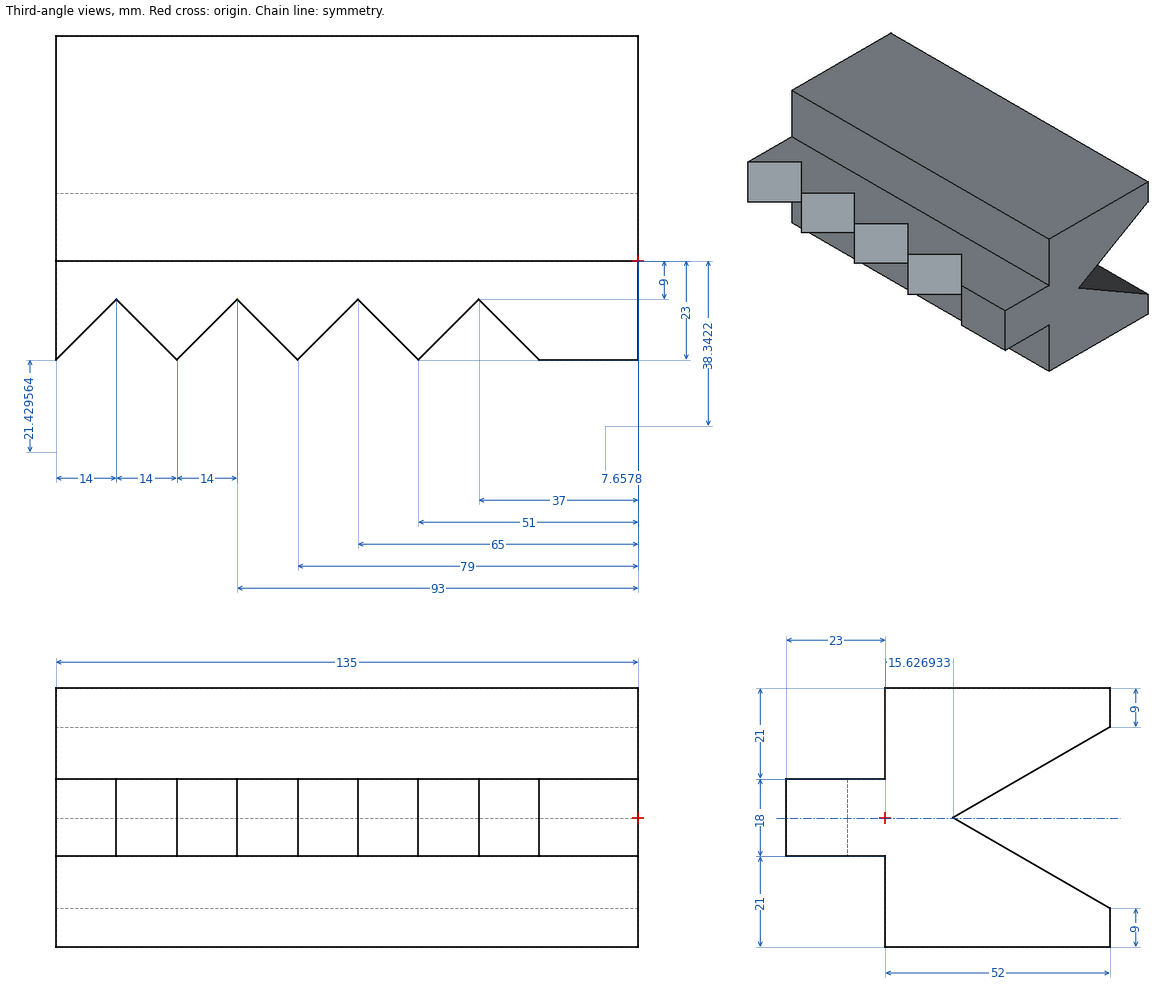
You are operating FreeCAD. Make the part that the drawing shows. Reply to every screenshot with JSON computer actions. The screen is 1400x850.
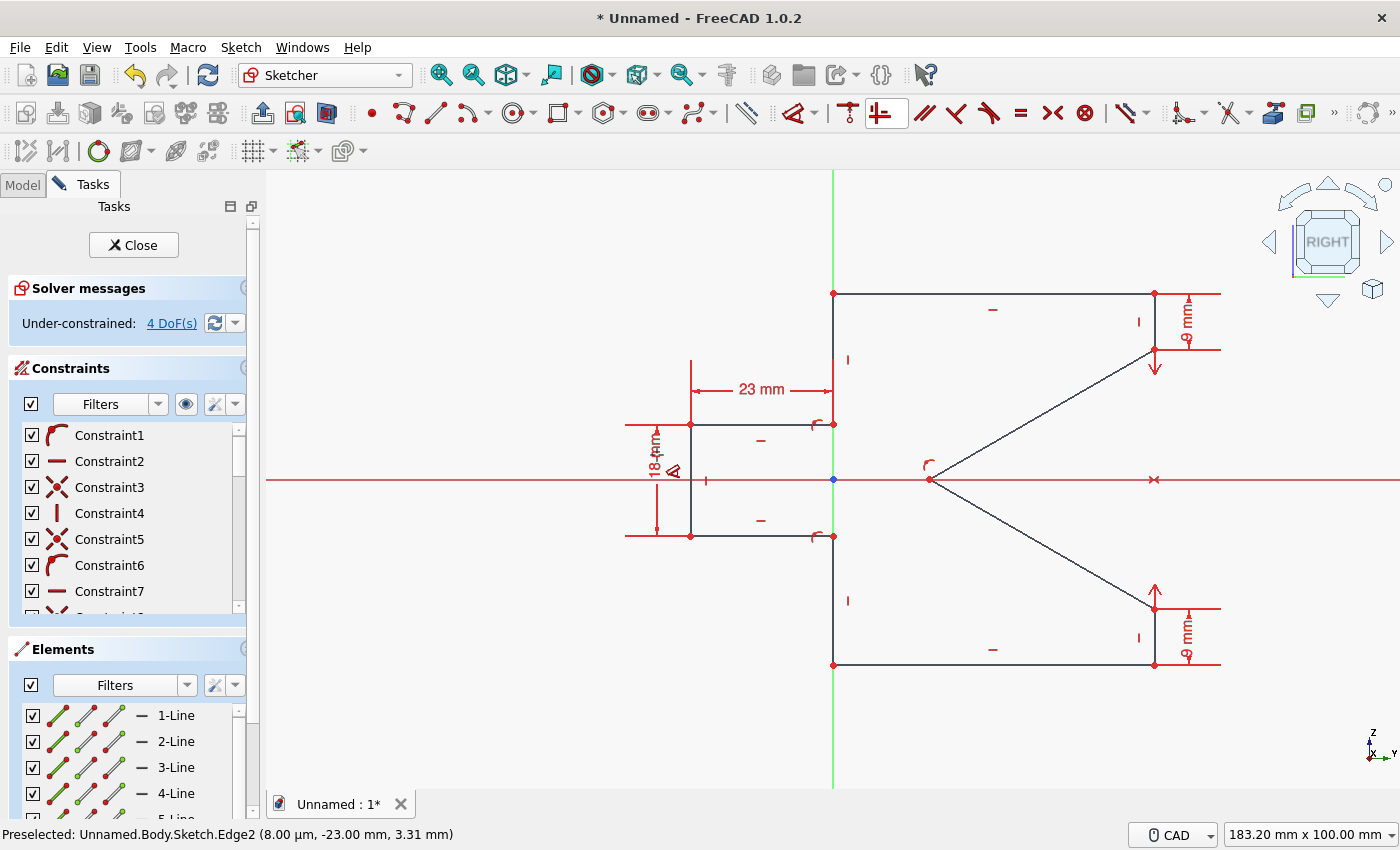
{"action": "left_click", "coordinate": [833, 575]}
{"action": "left_click", "coordinate": [799, 601]}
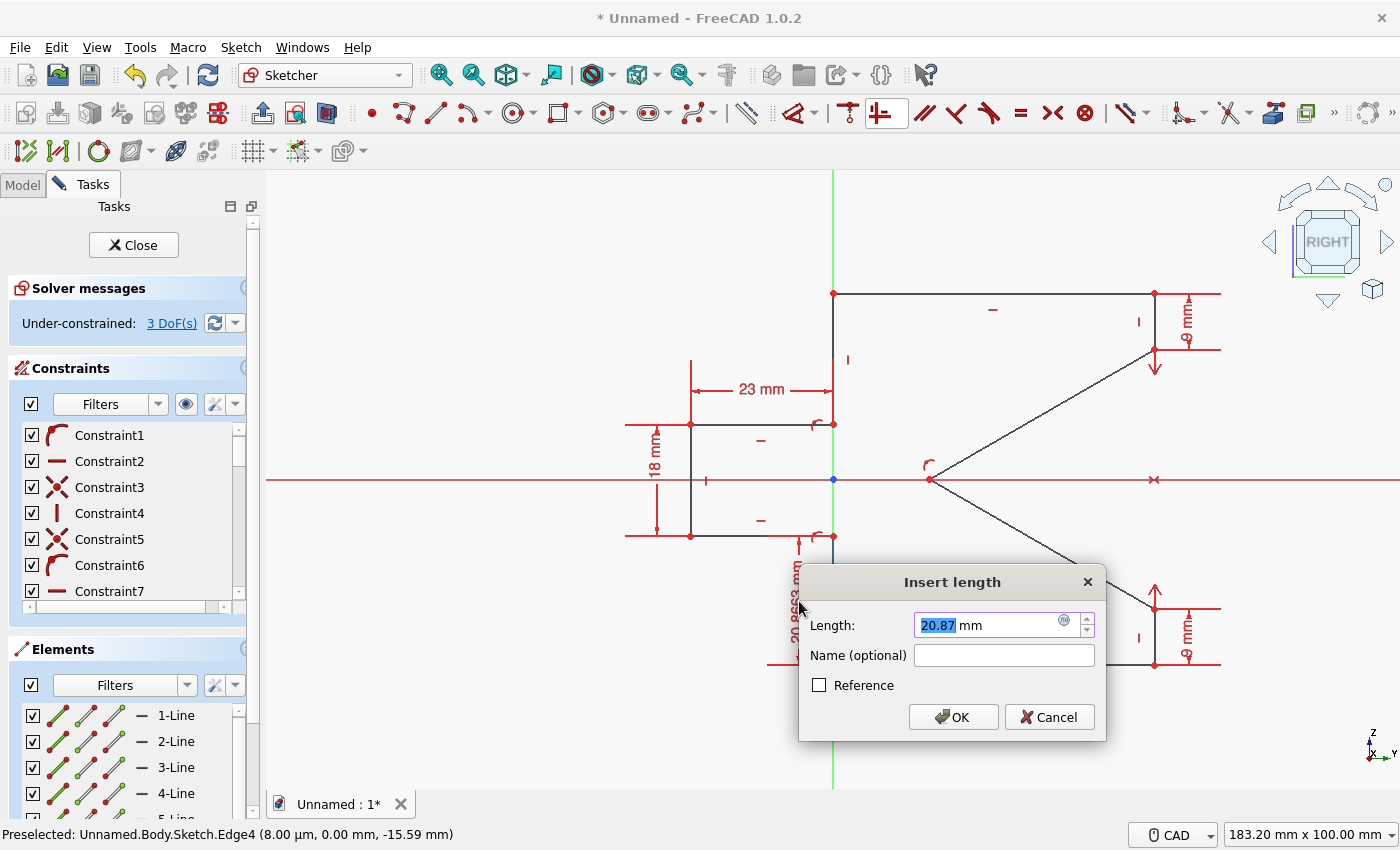
{"action": "type", "text": "21"}
{"action": "key", "text": "Return"}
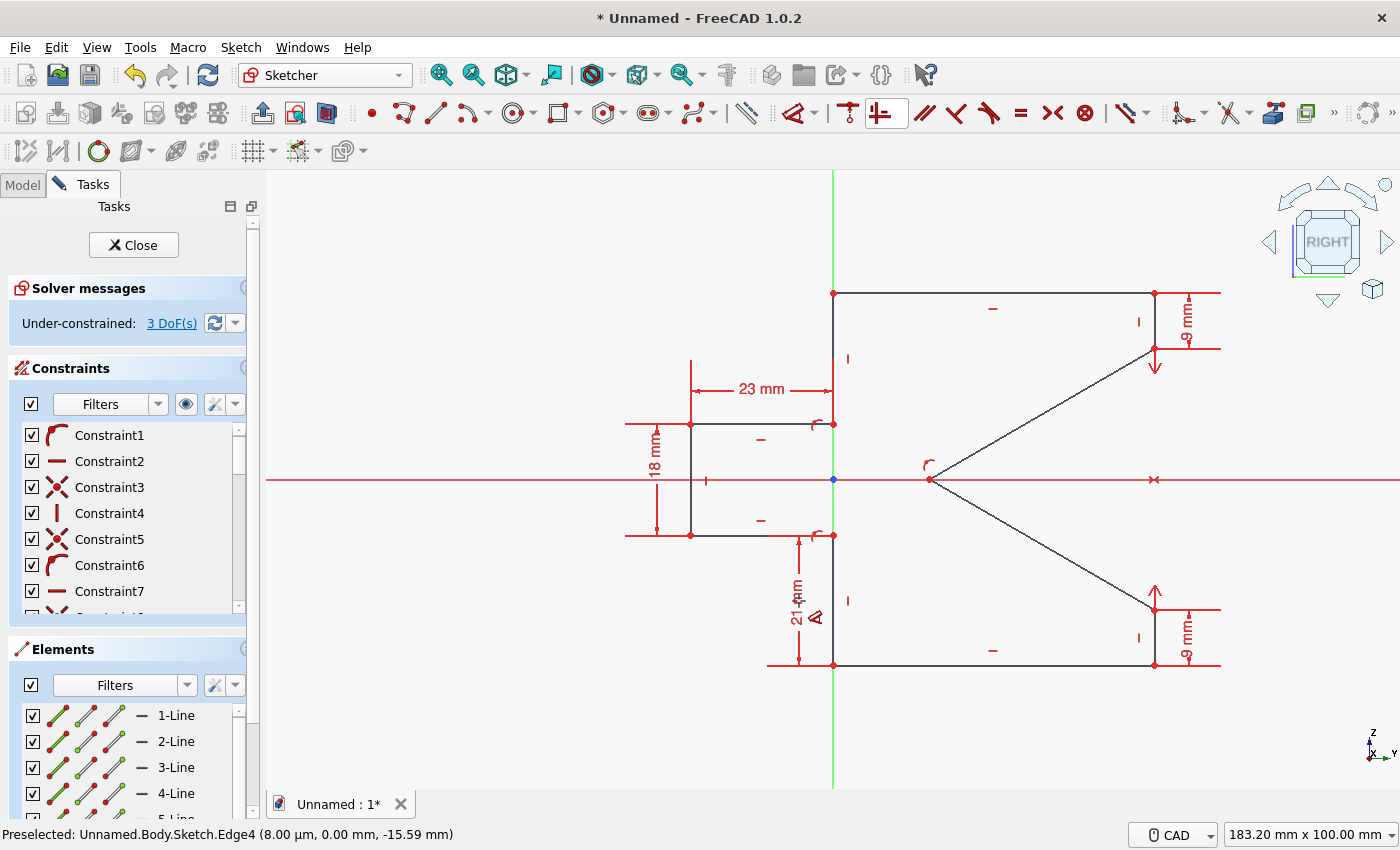
{"action": "left_click", "coordinate": [930, 666]}
{"action": "left_click", "coordinate": [994, 700]}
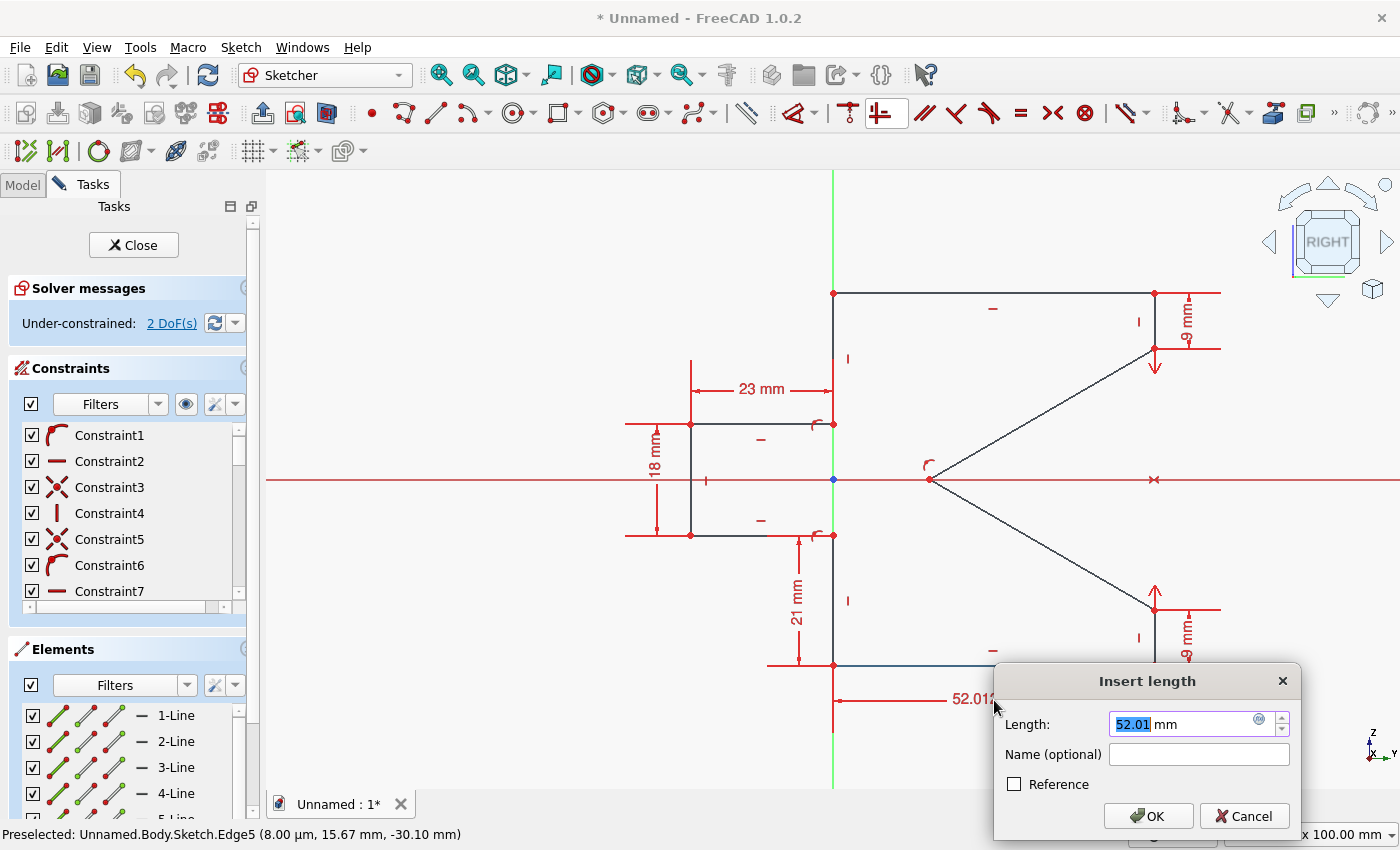
{"action": "type", "text": "52"}
{"action": "key", "text": "Return"}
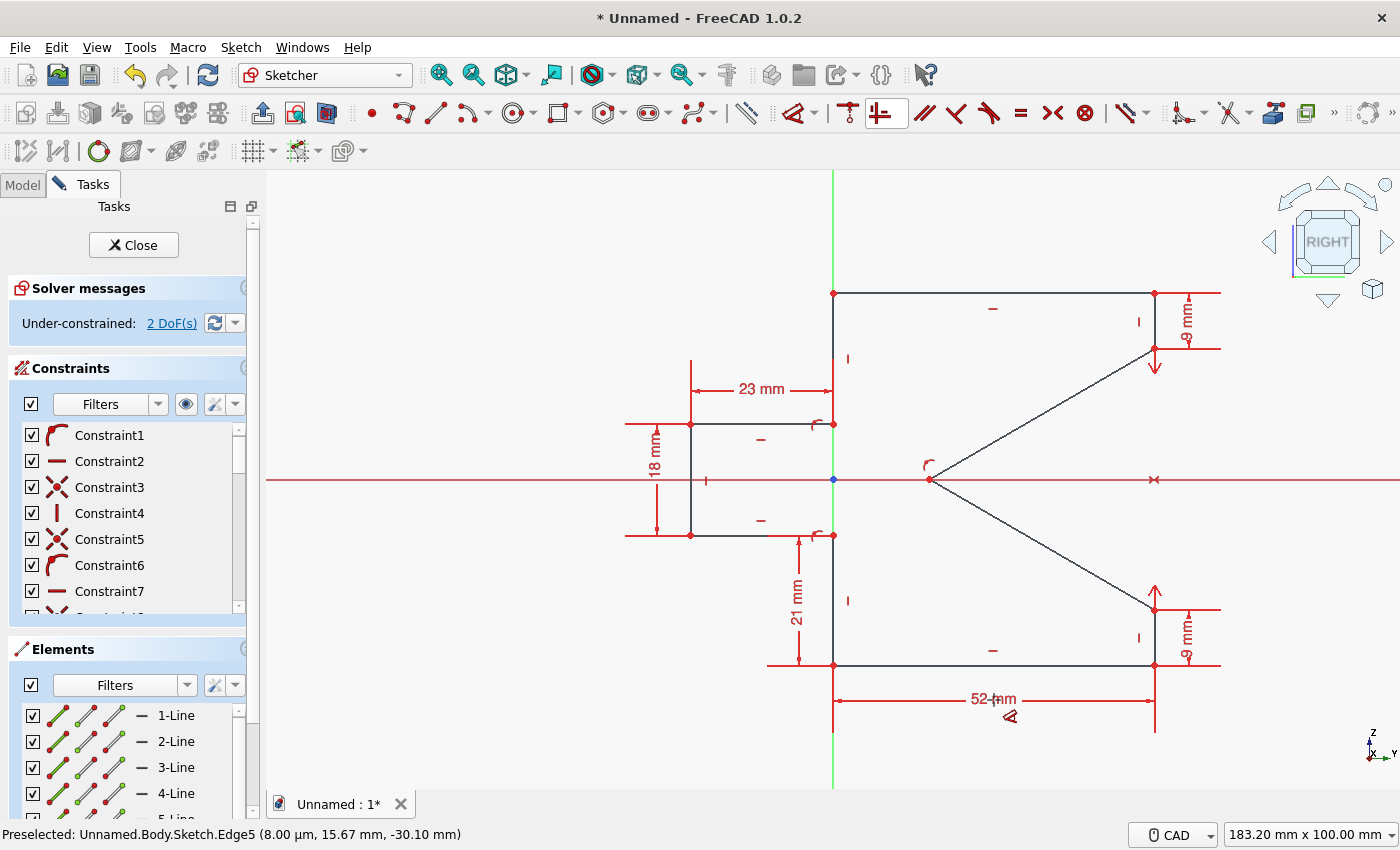
{"action": "left_click", "coordinate": [833, 333]}
{"action": "left_click", "coordinate": [799, 359]}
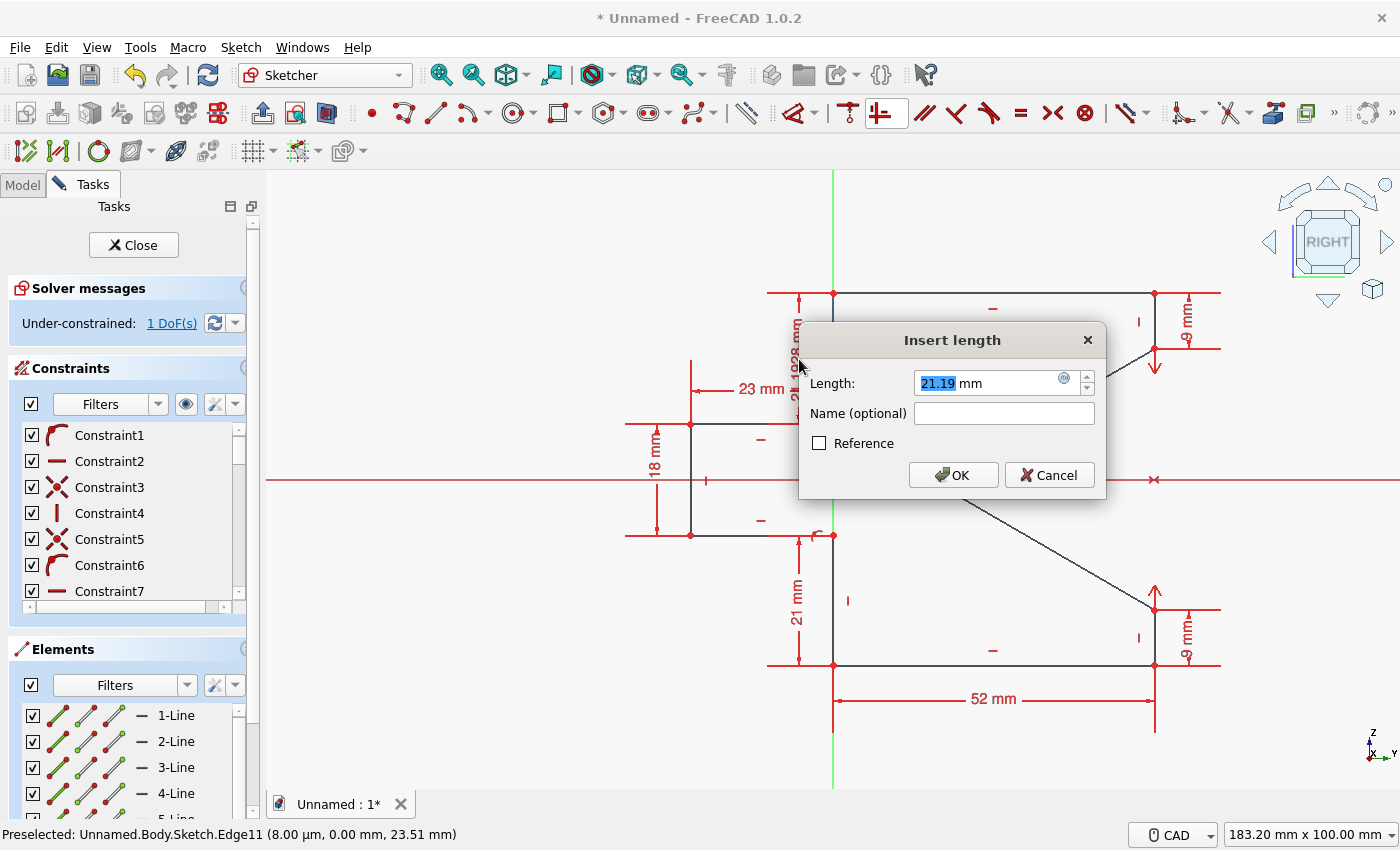
{"action": "type", "text": "21"}
{"action": "key", "text": "Return"}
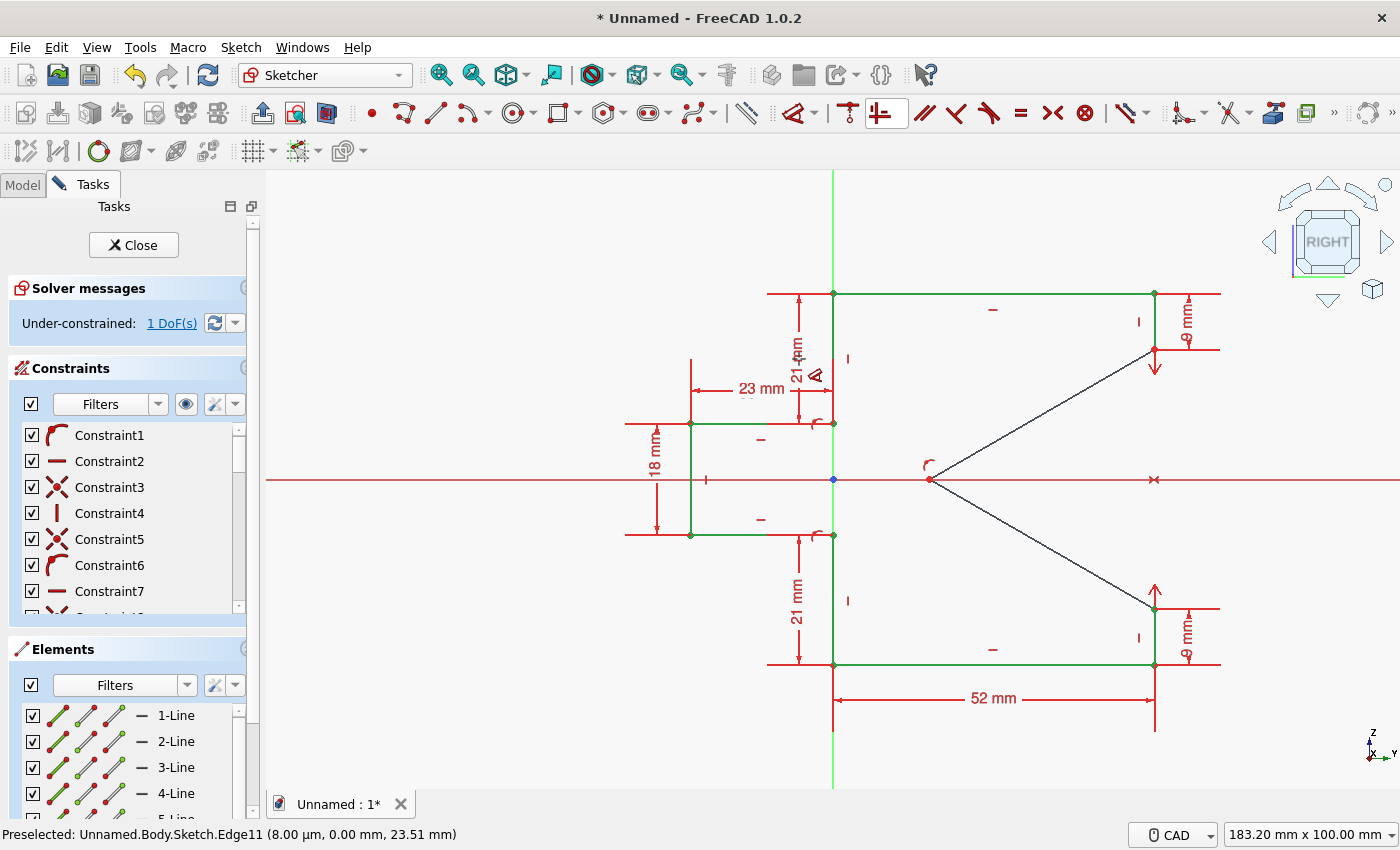
{"action": "left_click", "coordinate": [930, 480]}
{"action": "left_click", "coordinate": [881, 514]}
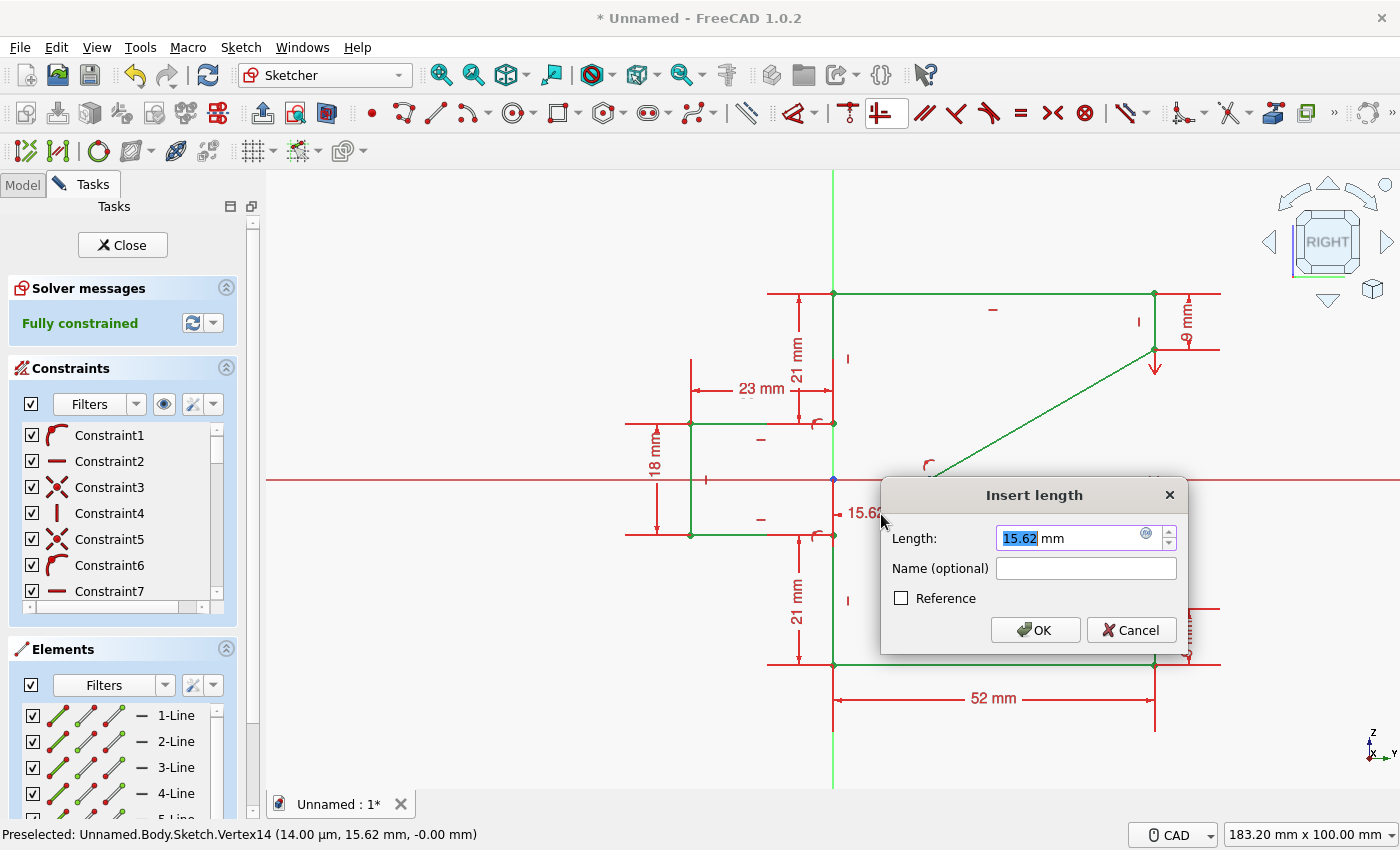
{"action": "type", "text": "15.626933"}
{"action": "key", "text": "Return"}
{"action": "key", "text": "Escape"}